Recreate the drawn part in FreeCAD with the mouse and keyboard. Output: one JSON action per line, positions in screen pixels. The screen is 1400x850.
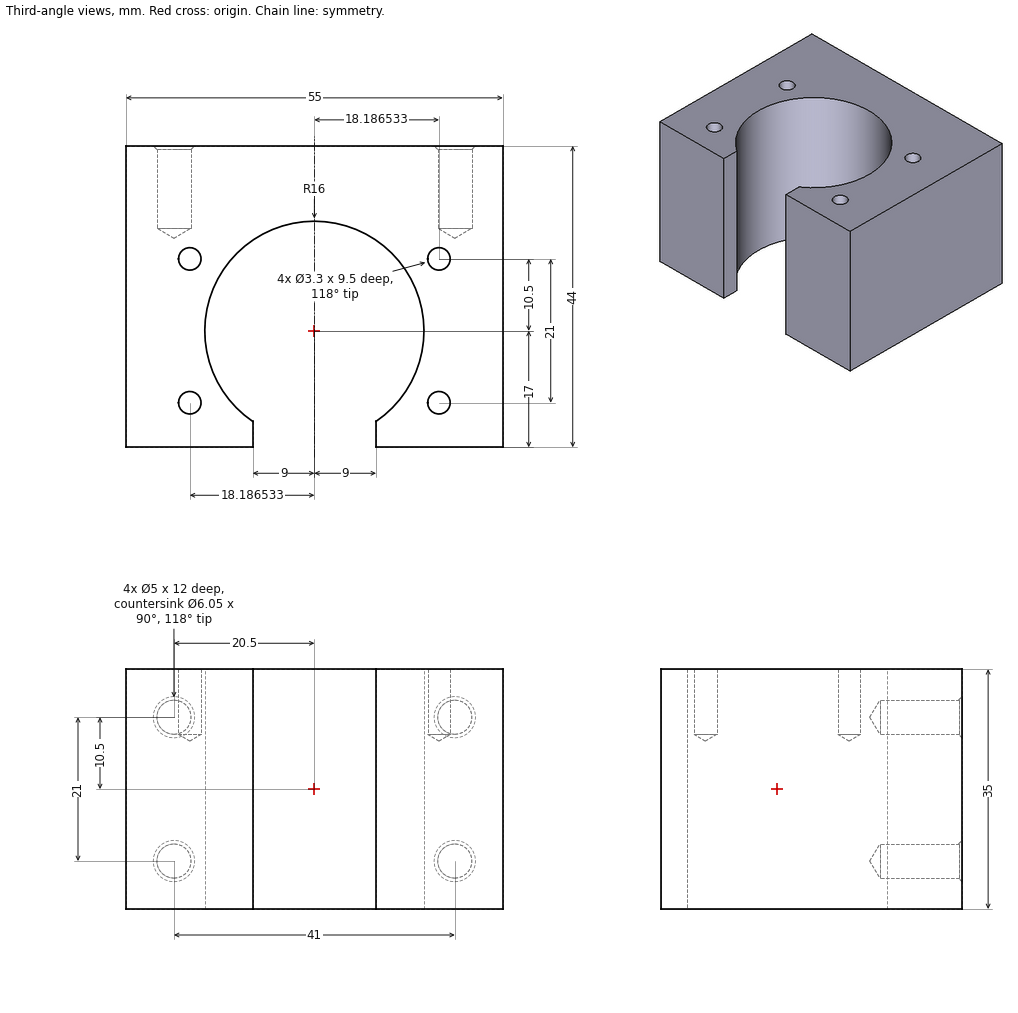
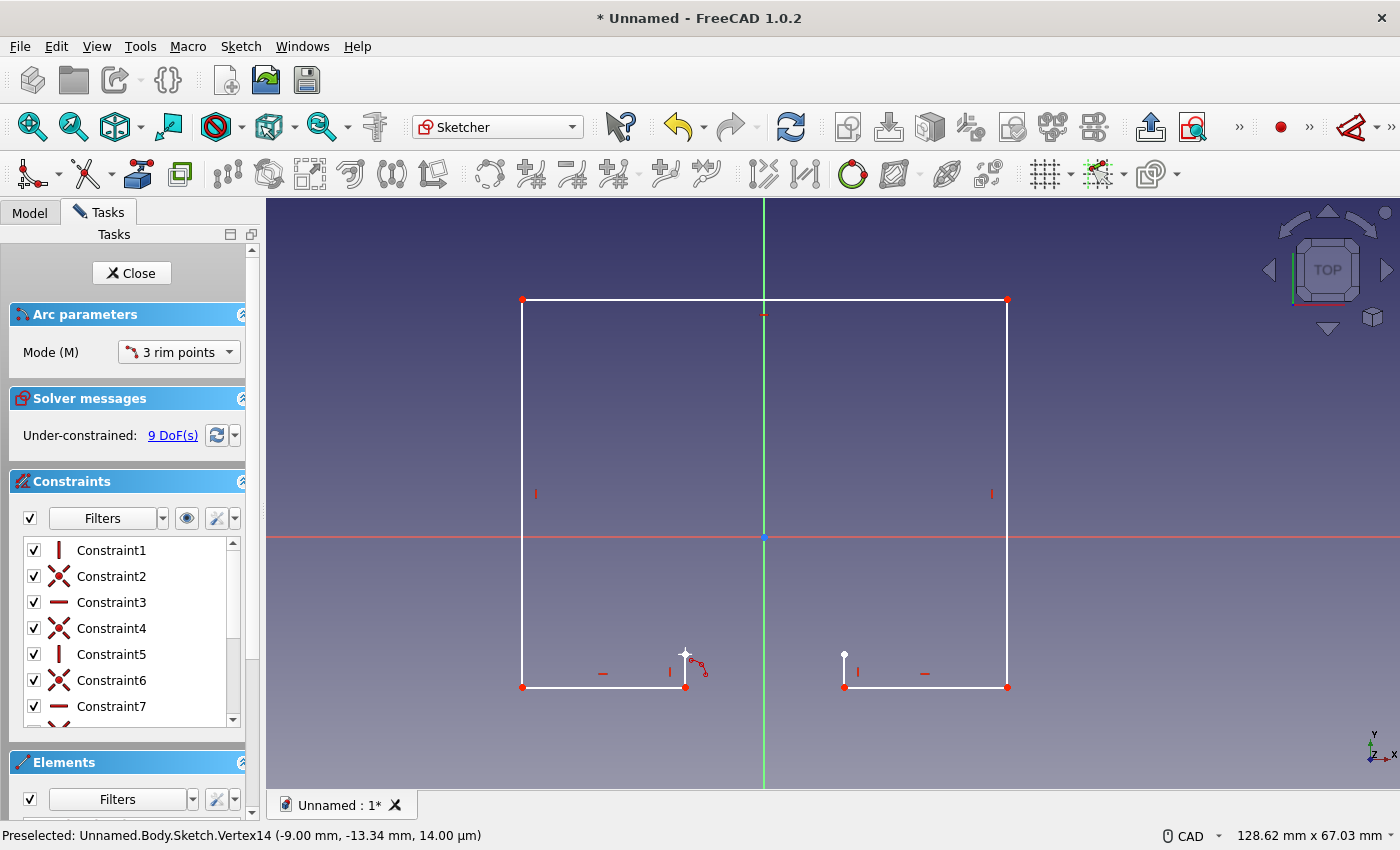
{"action": "left_click", "coordinate": [685, 655]}
{"action": "left_click", "coordinate": [844, 655]}
{"action": "left_click", "coordinate": [833, 414]}
{"action": "key", "text": "Escape"}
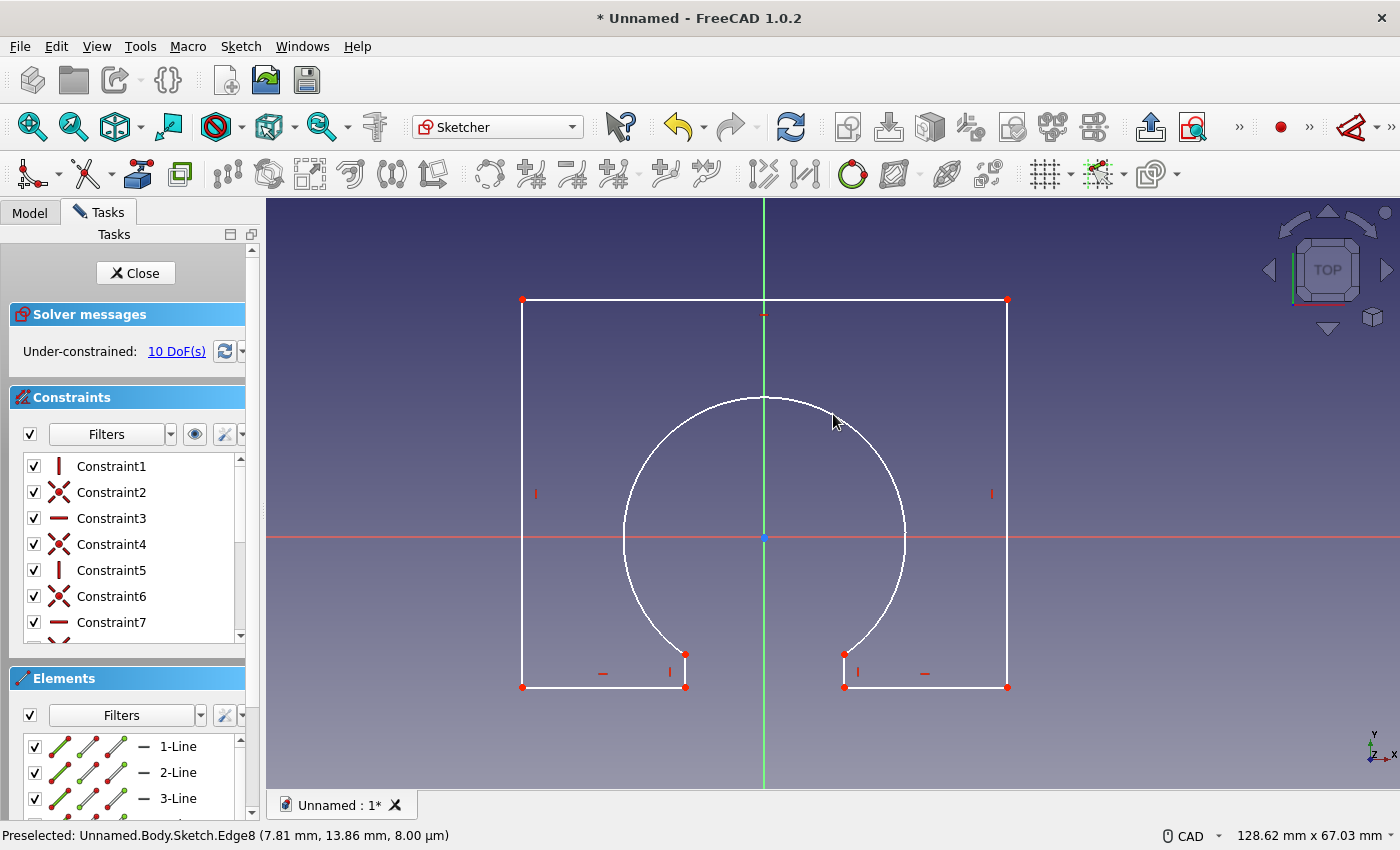
{"action": "left_click_drag", "start_coordinate": [754, 527], "coordinate": [774, 548]}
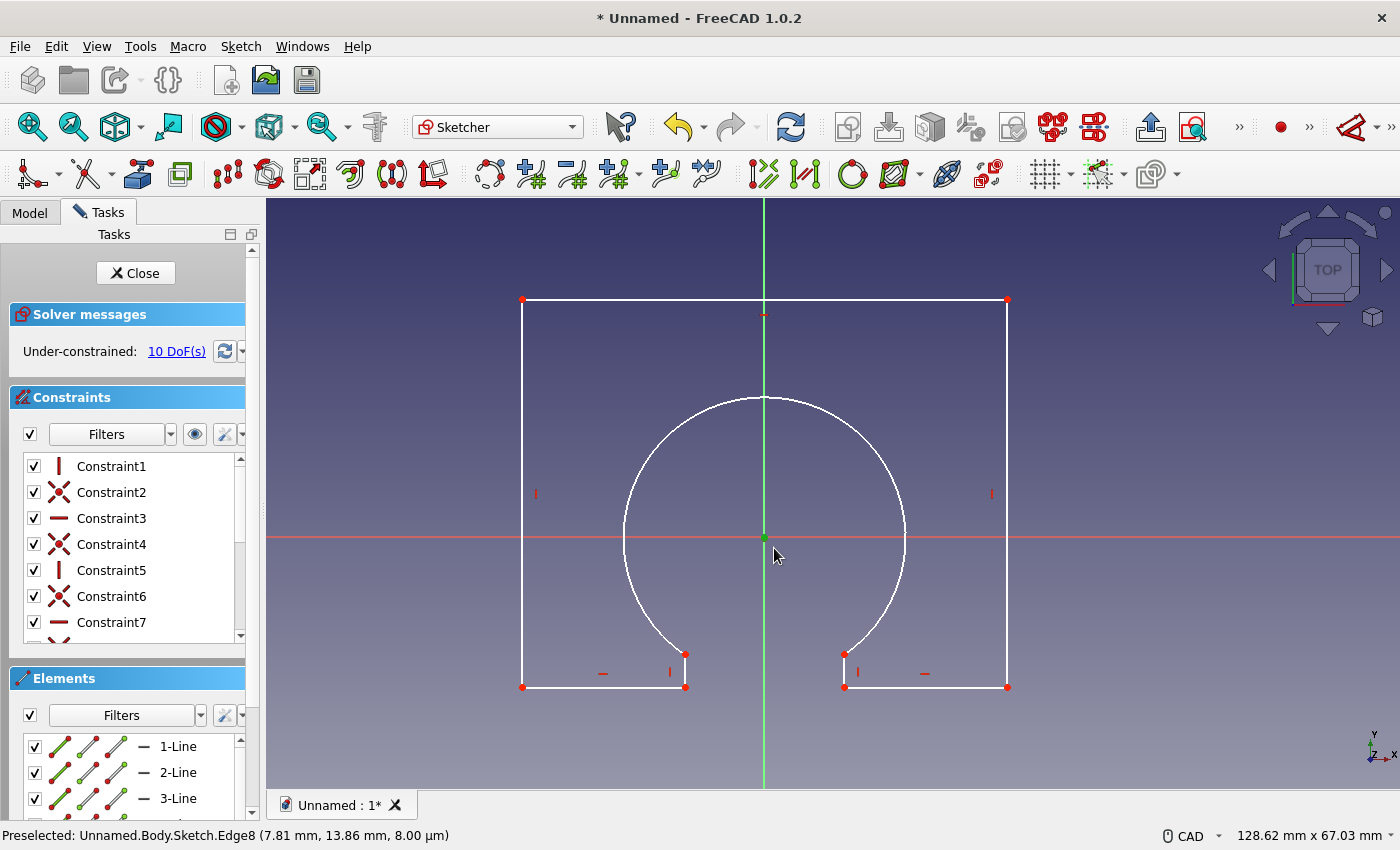
{"action": "key", "text": "c"}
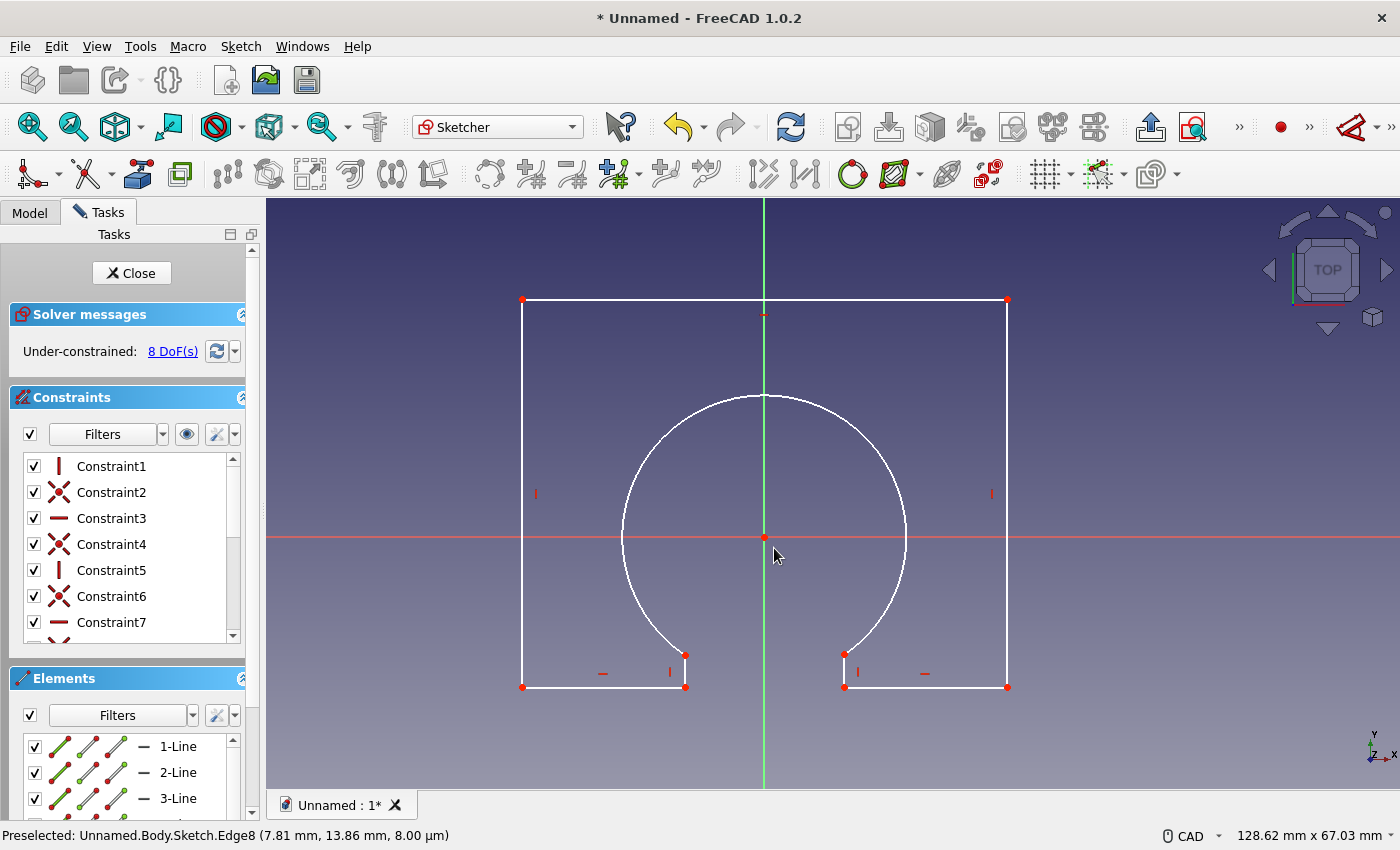
{"action": "left_click", "coordinate": [1007, 688]}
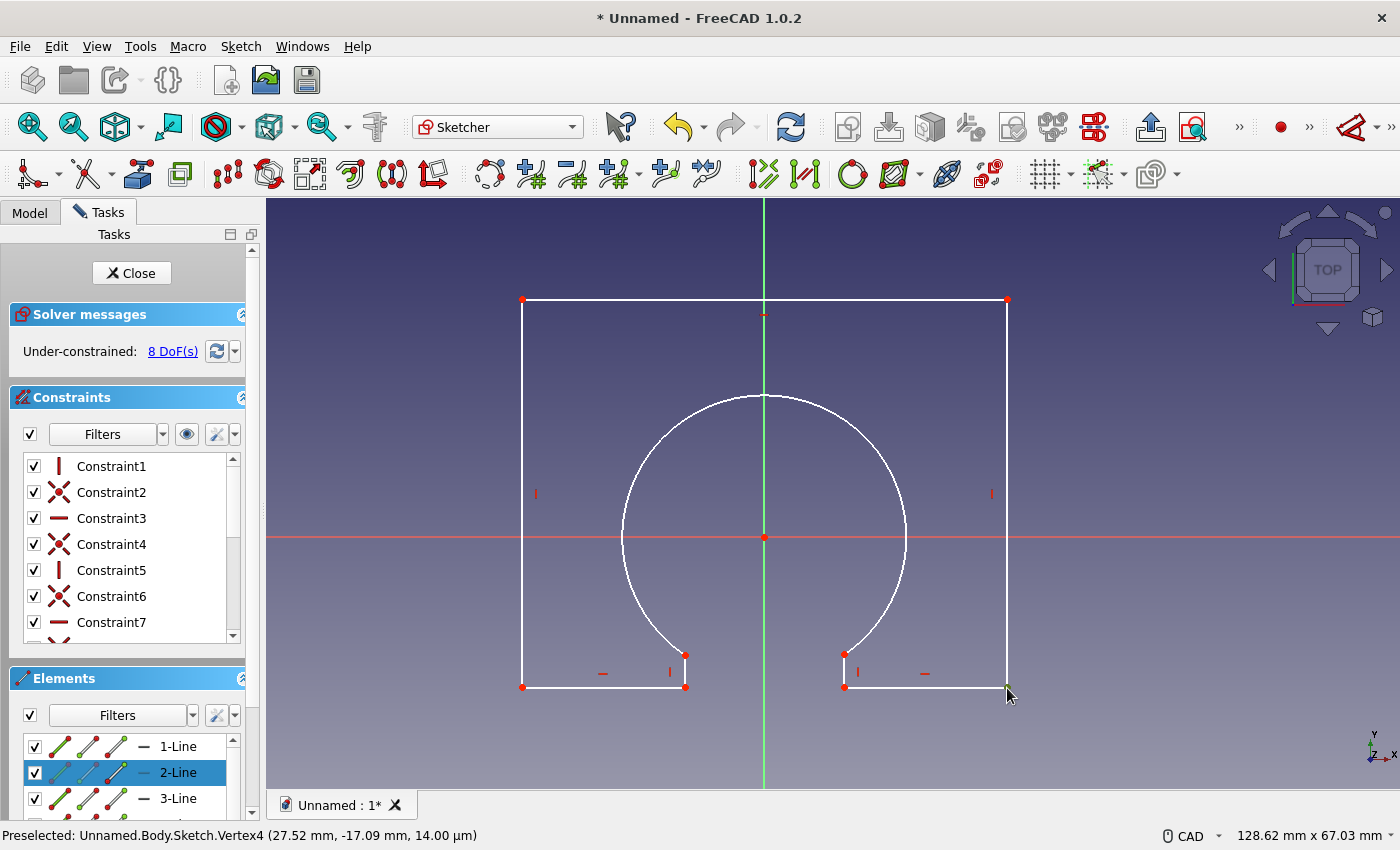
{"action": "left_click", "coordinate": [522, 688]}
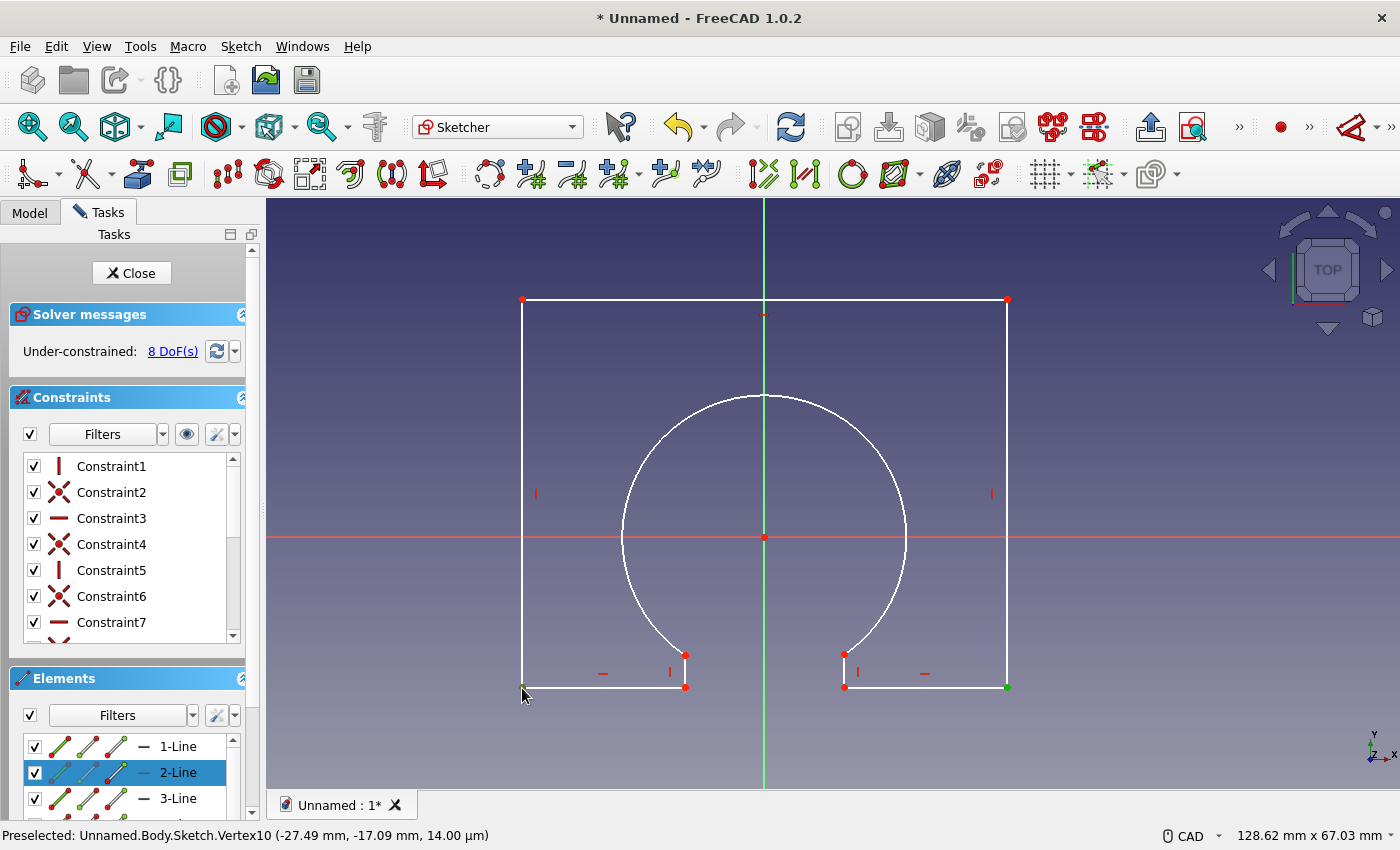
{"action": "left_click", "coordinate": [764, 723]}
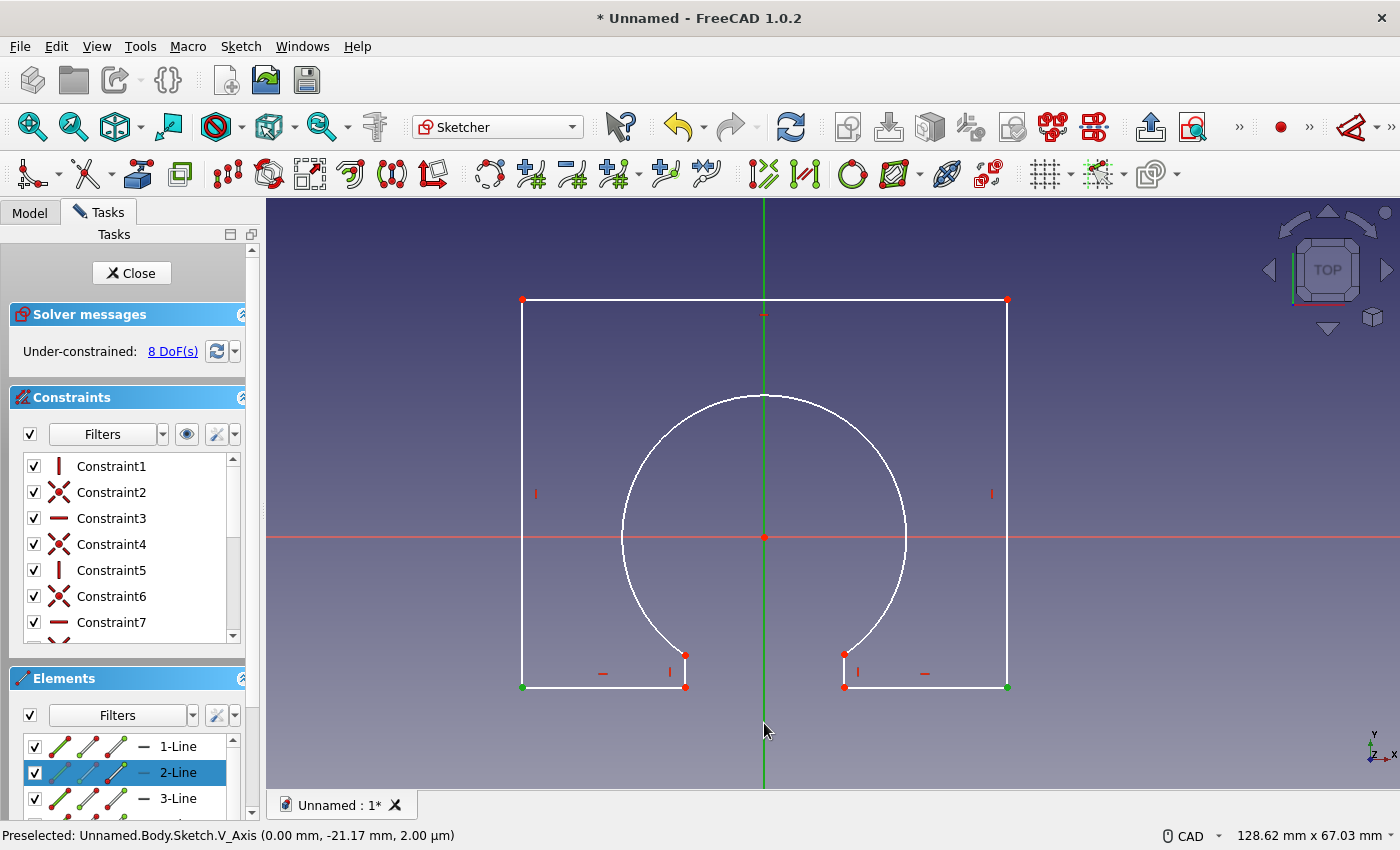
{"action": "key", "text": "s"}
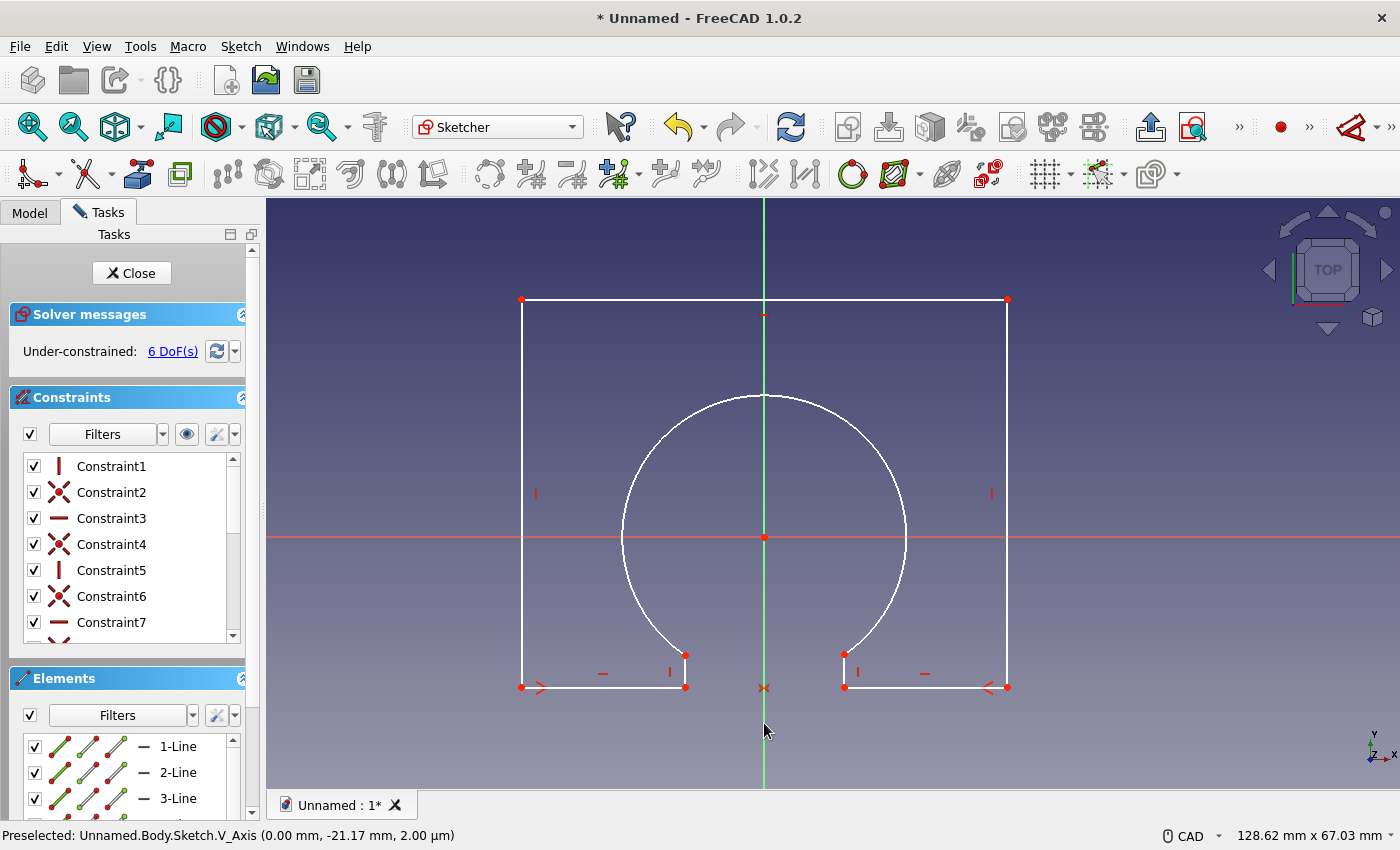
{"action": "left_click", "coordinate": [1350, 128]}